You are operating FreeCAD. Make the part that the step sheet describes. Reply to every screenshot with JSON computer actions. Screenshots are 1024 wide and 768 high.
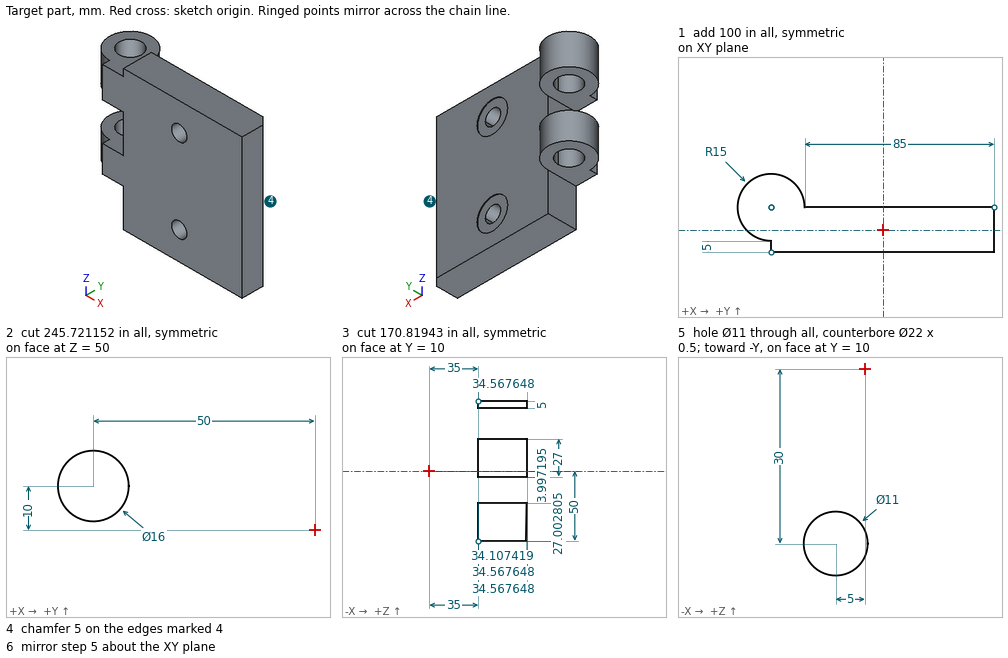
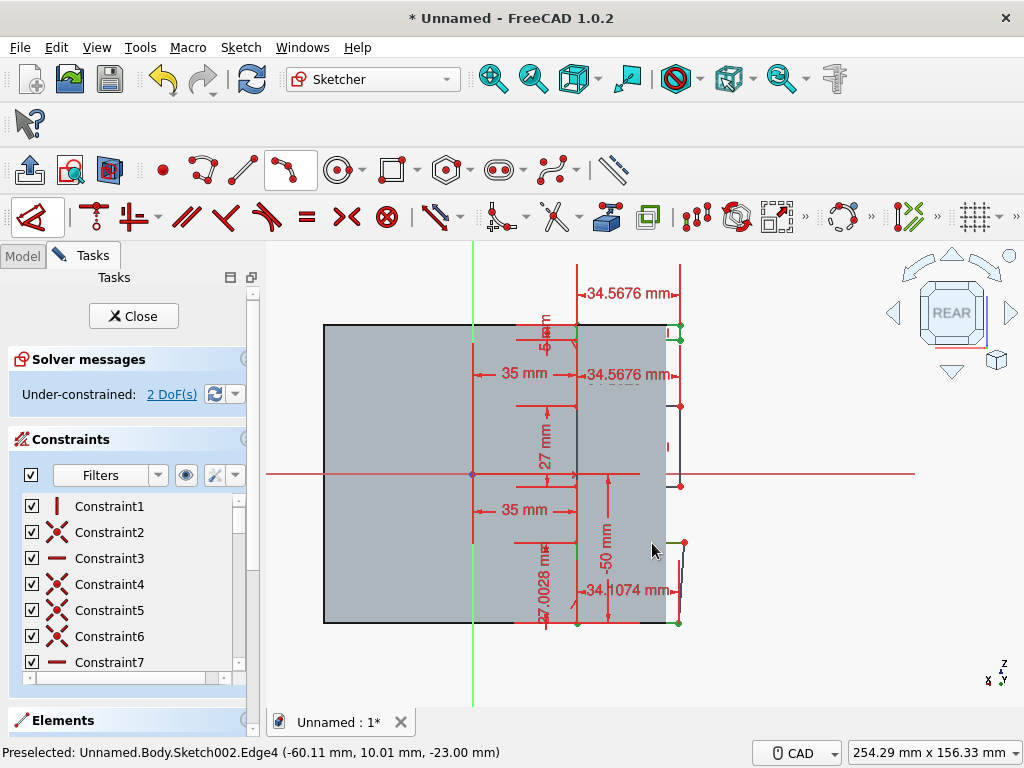
{"action": "key", "text": "l"}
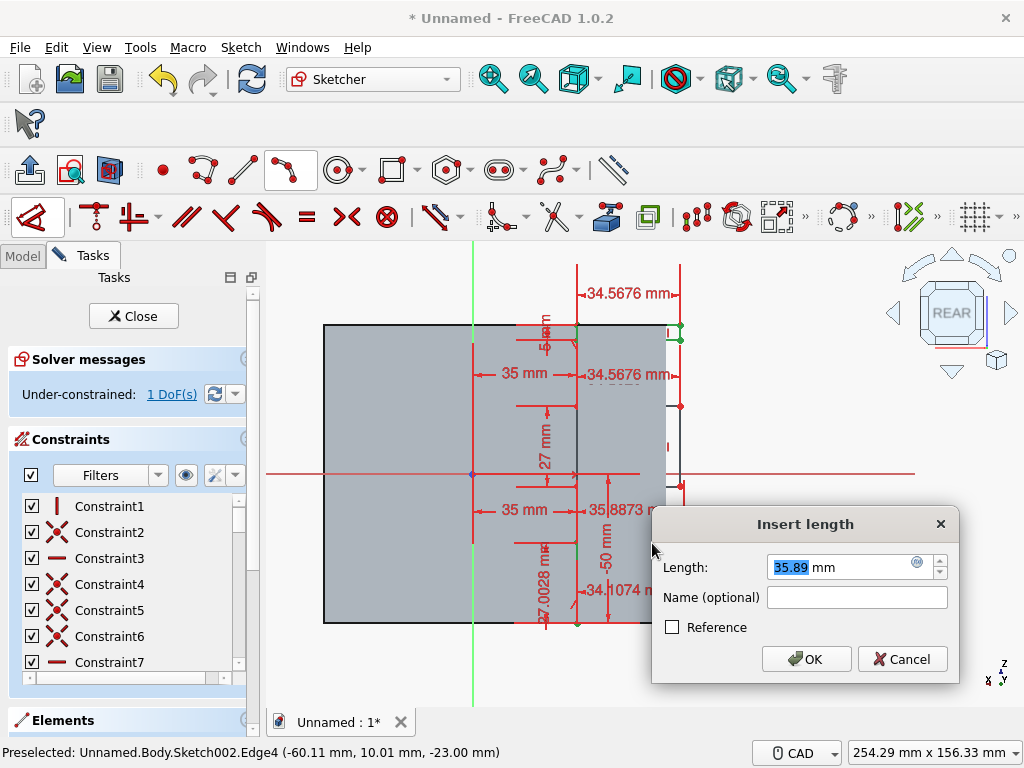
{"action": "type", "text": "34.567648"}
{"action": "key", "text": "Return"}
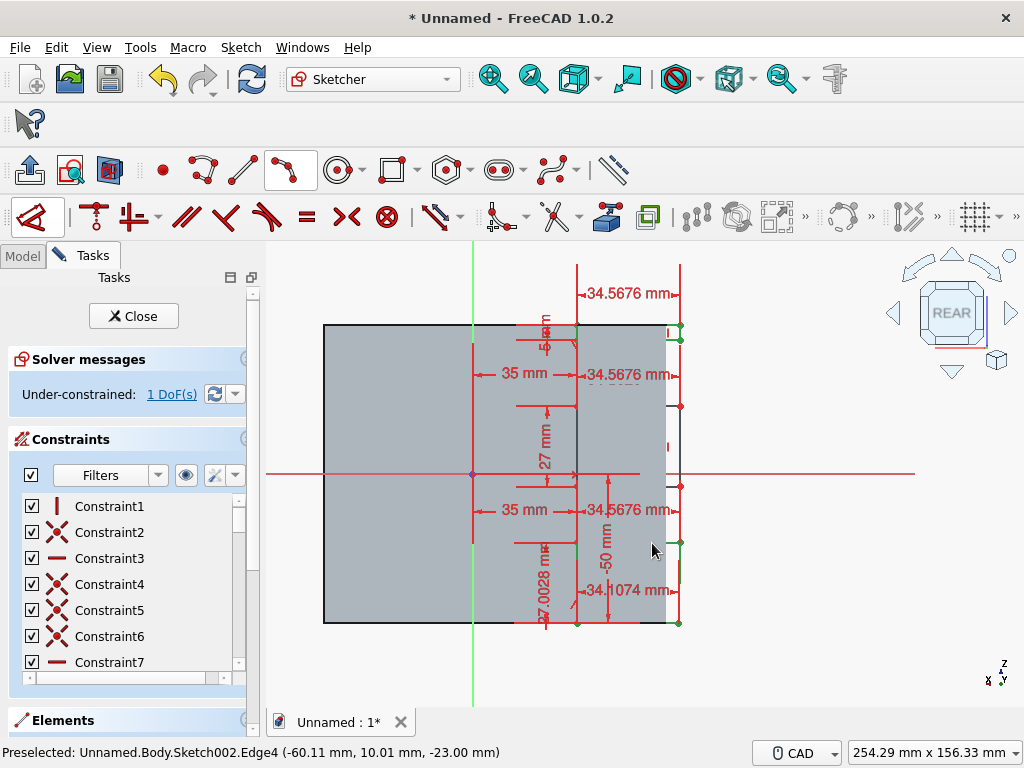
{"action": "scroll", "coordinate": [577, 487], "scroll_direction": "up", "scroll_amount": 7}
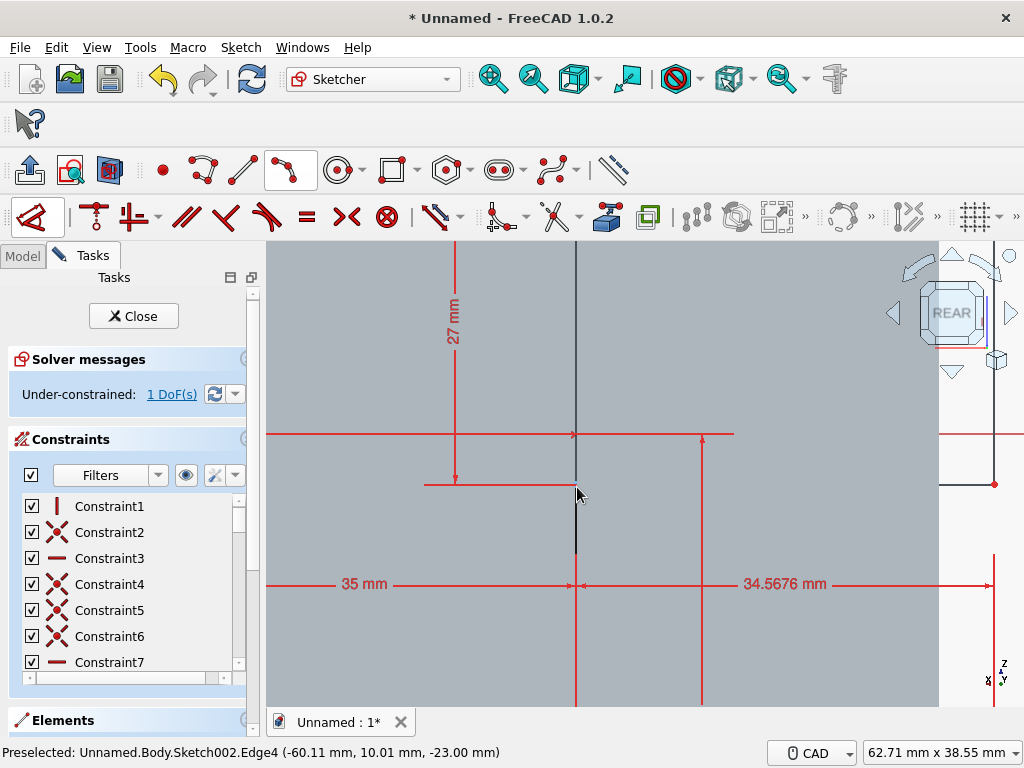
{"action": "left_click", "coordinate": [576, 485]}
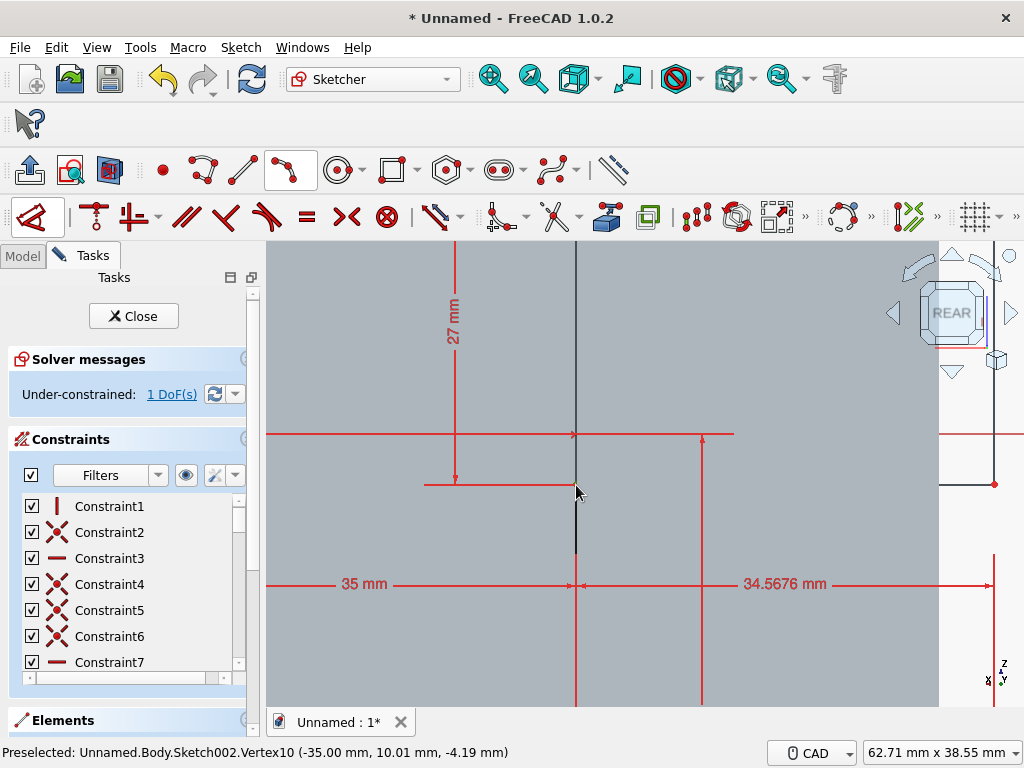
{"action": "left_click", "coordinate": [58, 218]}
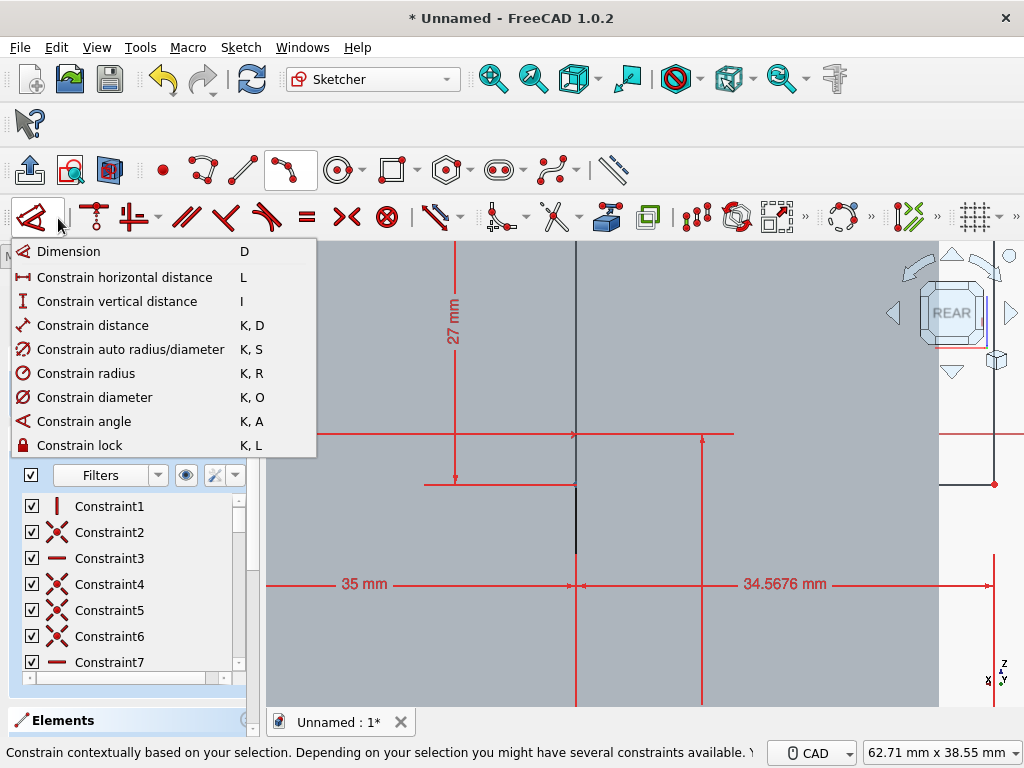
{"action": "left_click", "coordinate": [164, 301]}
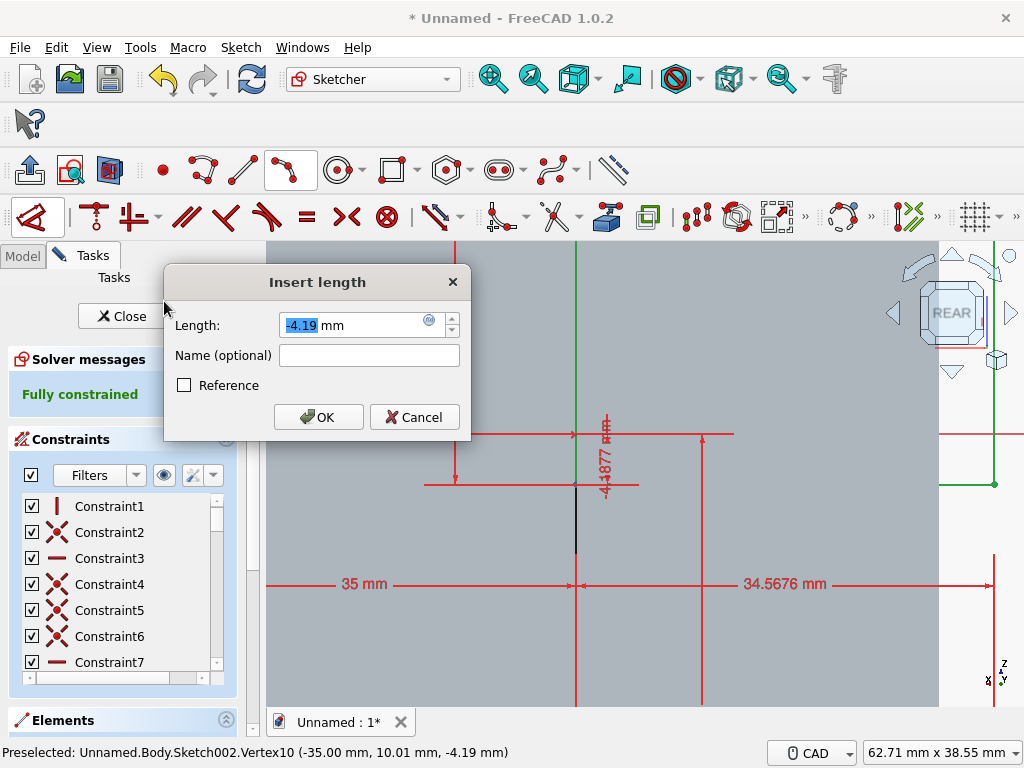
{"action": "type", "text": "-3.997195"}
{"action": "key", "text": "Return"}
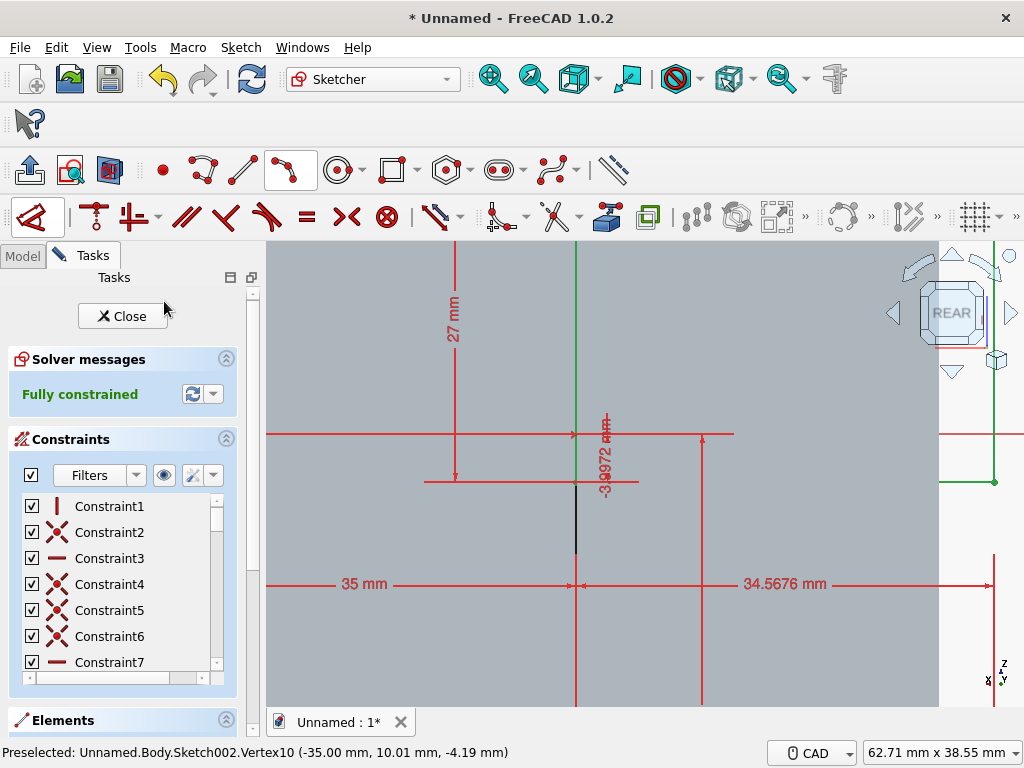
{"action": "left_click", "coordinate": [123, 316]}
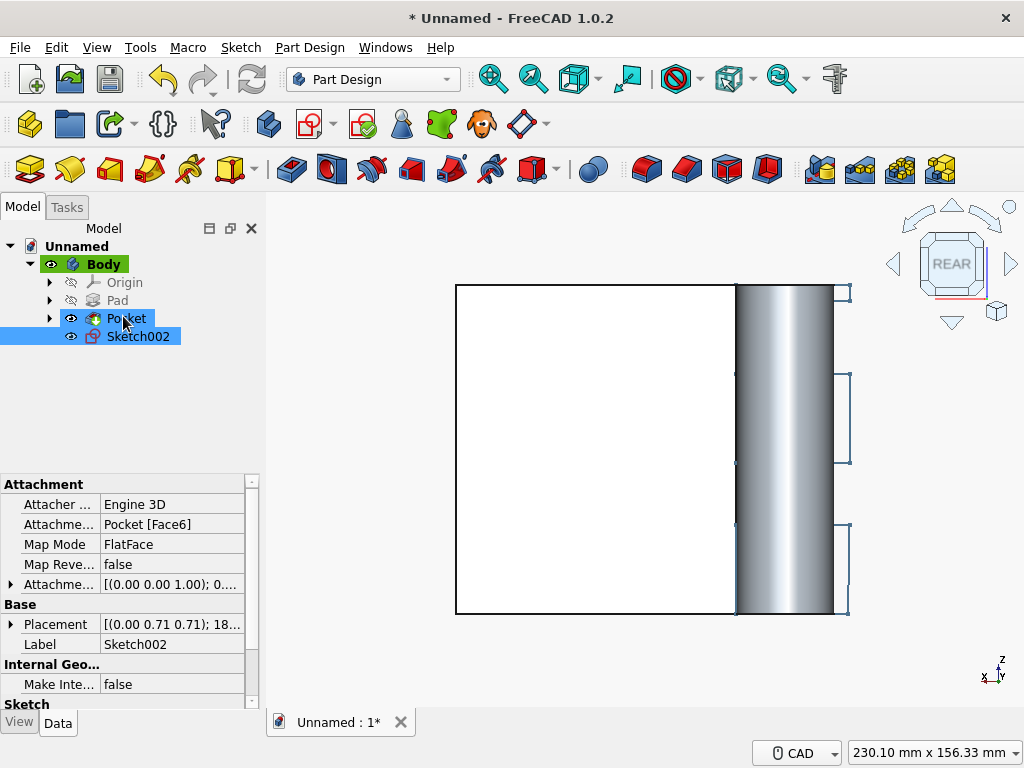
{"action": "left_click", "coordinate": [292, 170]}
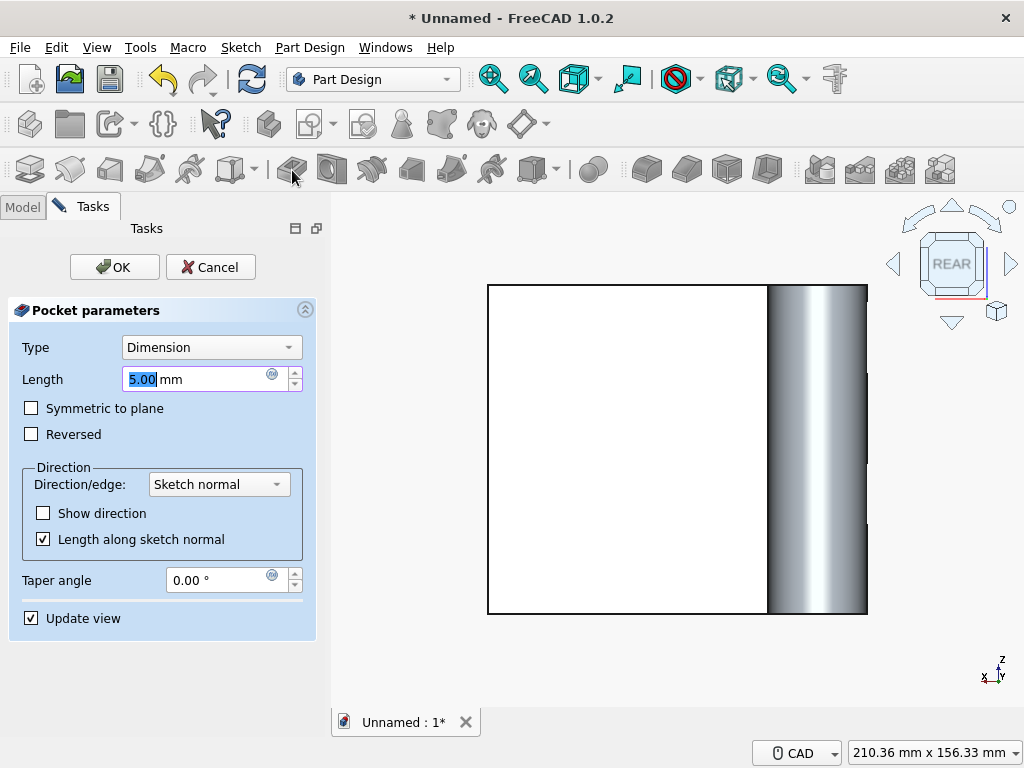
{"action": "type", "text": "170.81943"}
{"action": "key", "text": "Tab"}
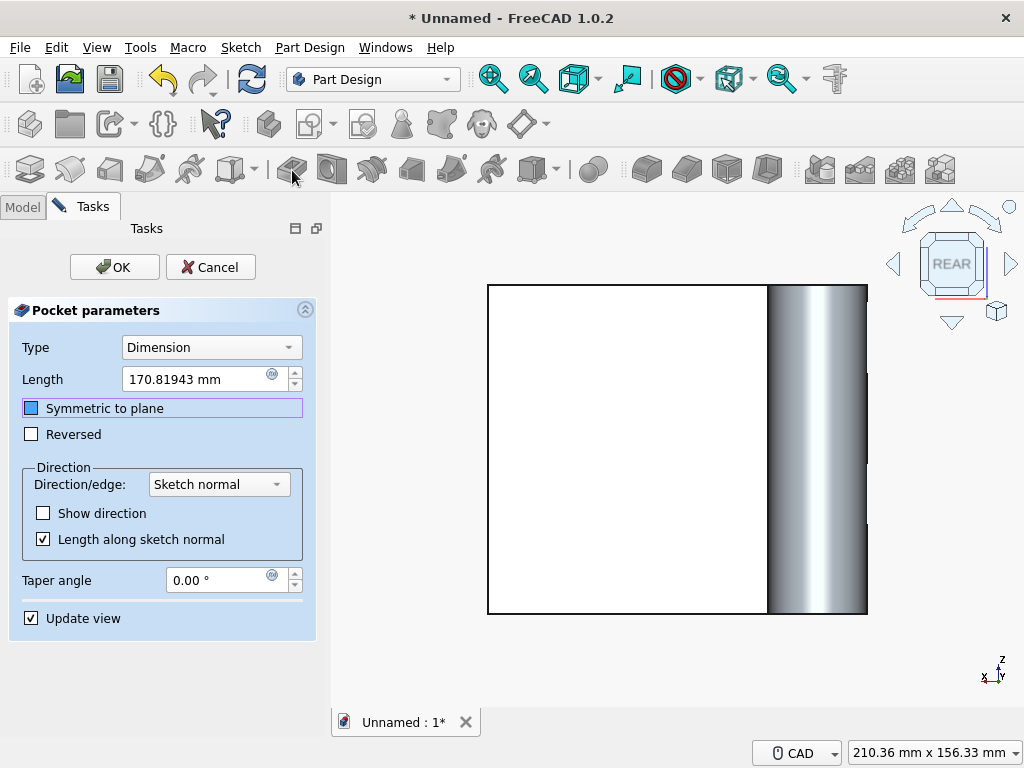
{"action": "left_click", "coordinate": [30, 408]}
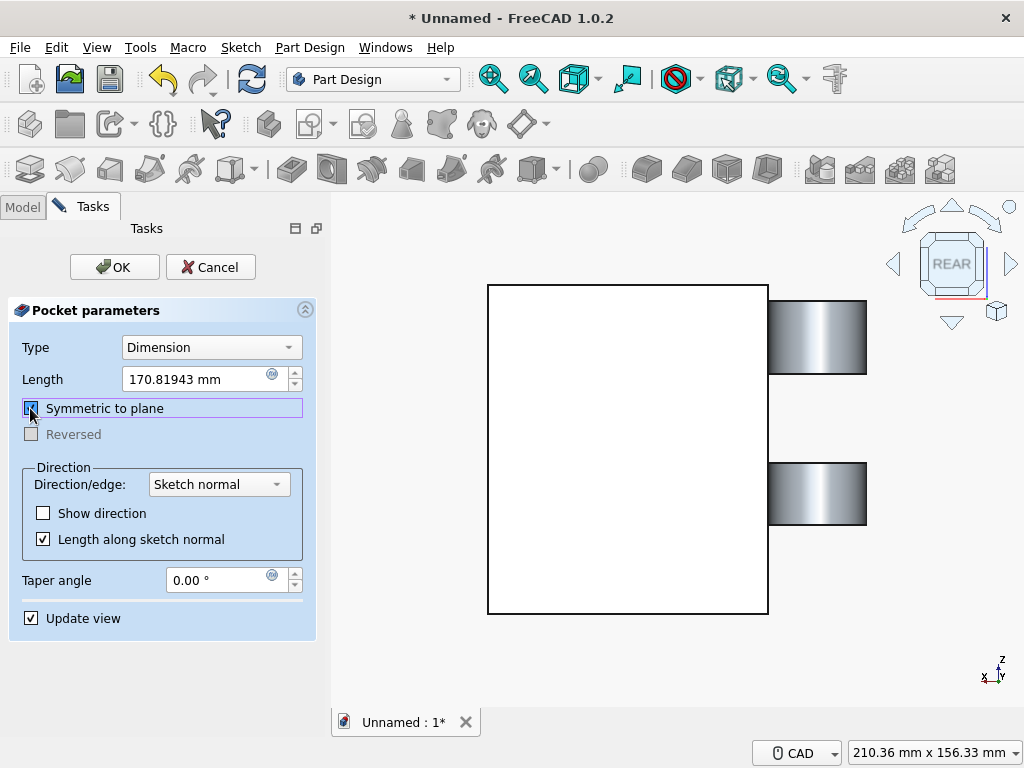
{"action": "left_click", "coordinate": [115, 267]}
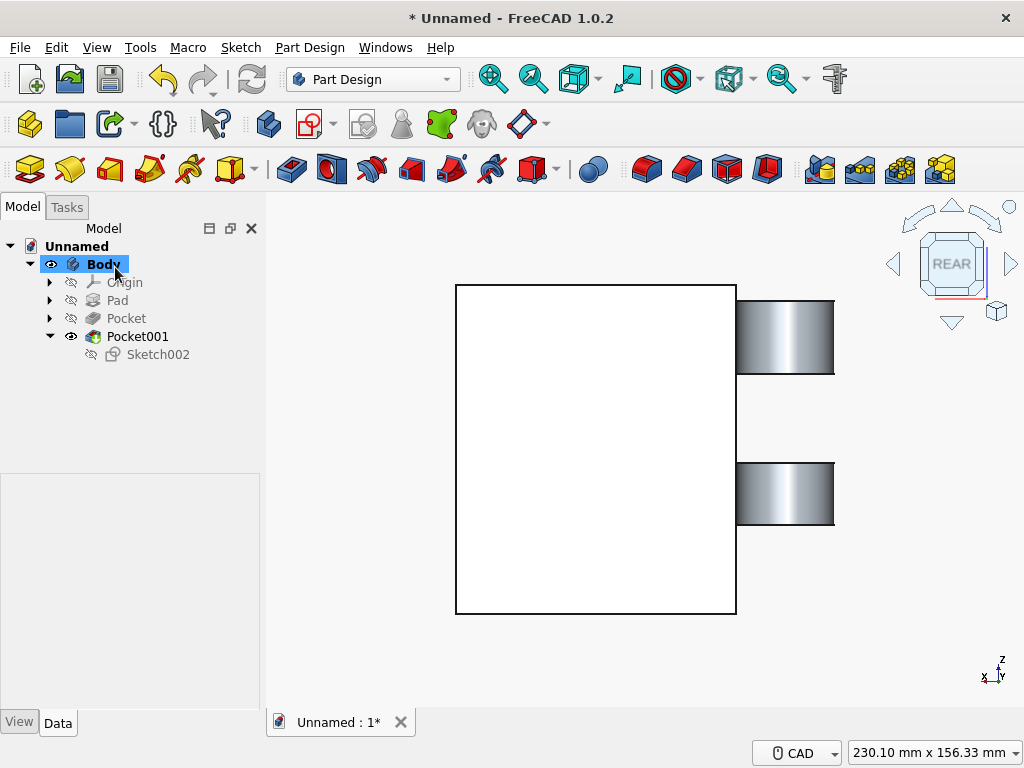
{"action": "key", "text": "0"}